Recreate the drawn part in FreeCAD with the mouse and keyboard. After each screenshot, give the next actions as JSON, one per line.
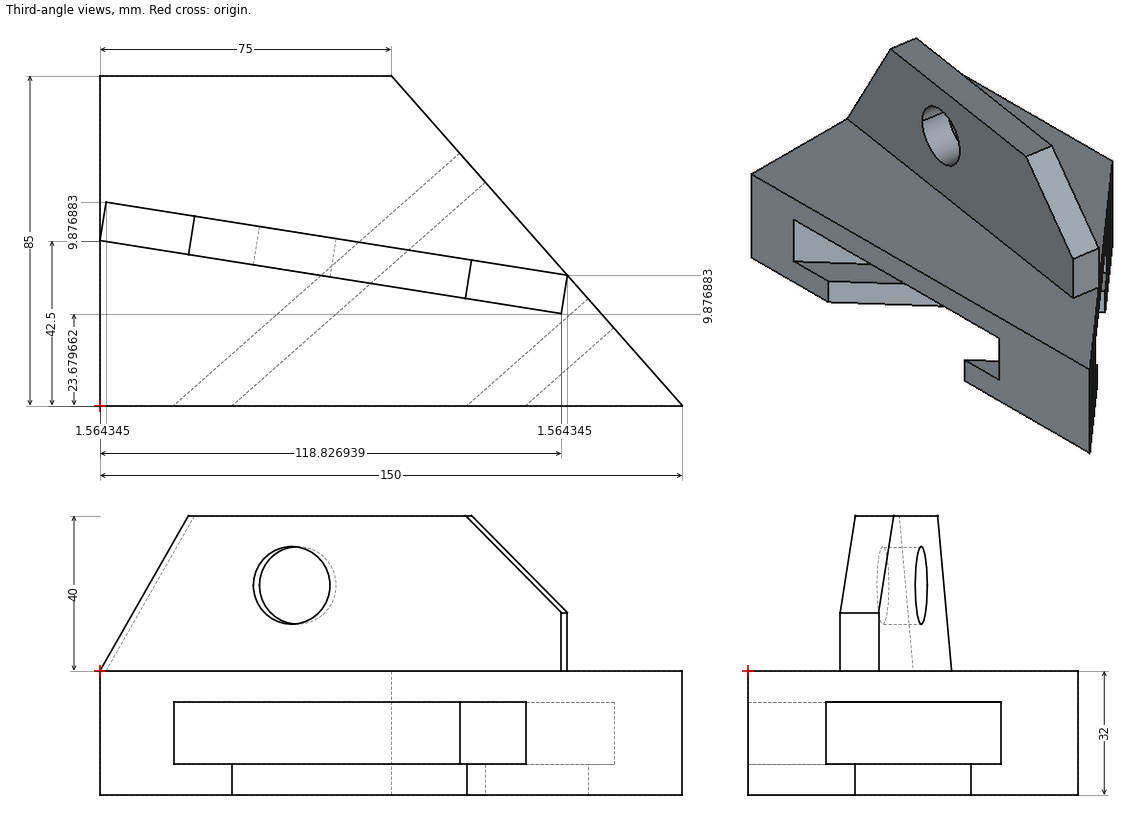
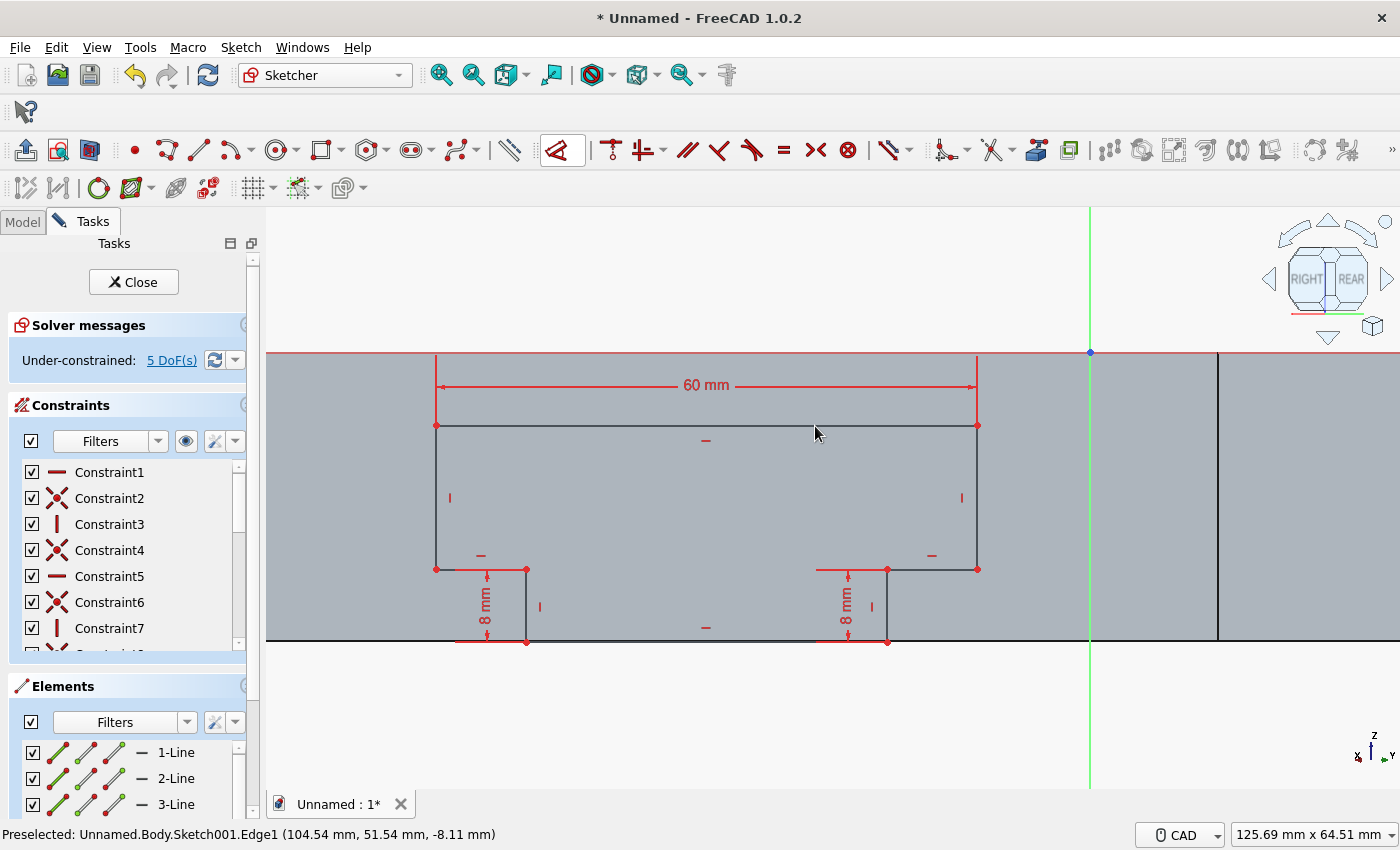
{"action": "left_click", "coordinate": [436, 469]}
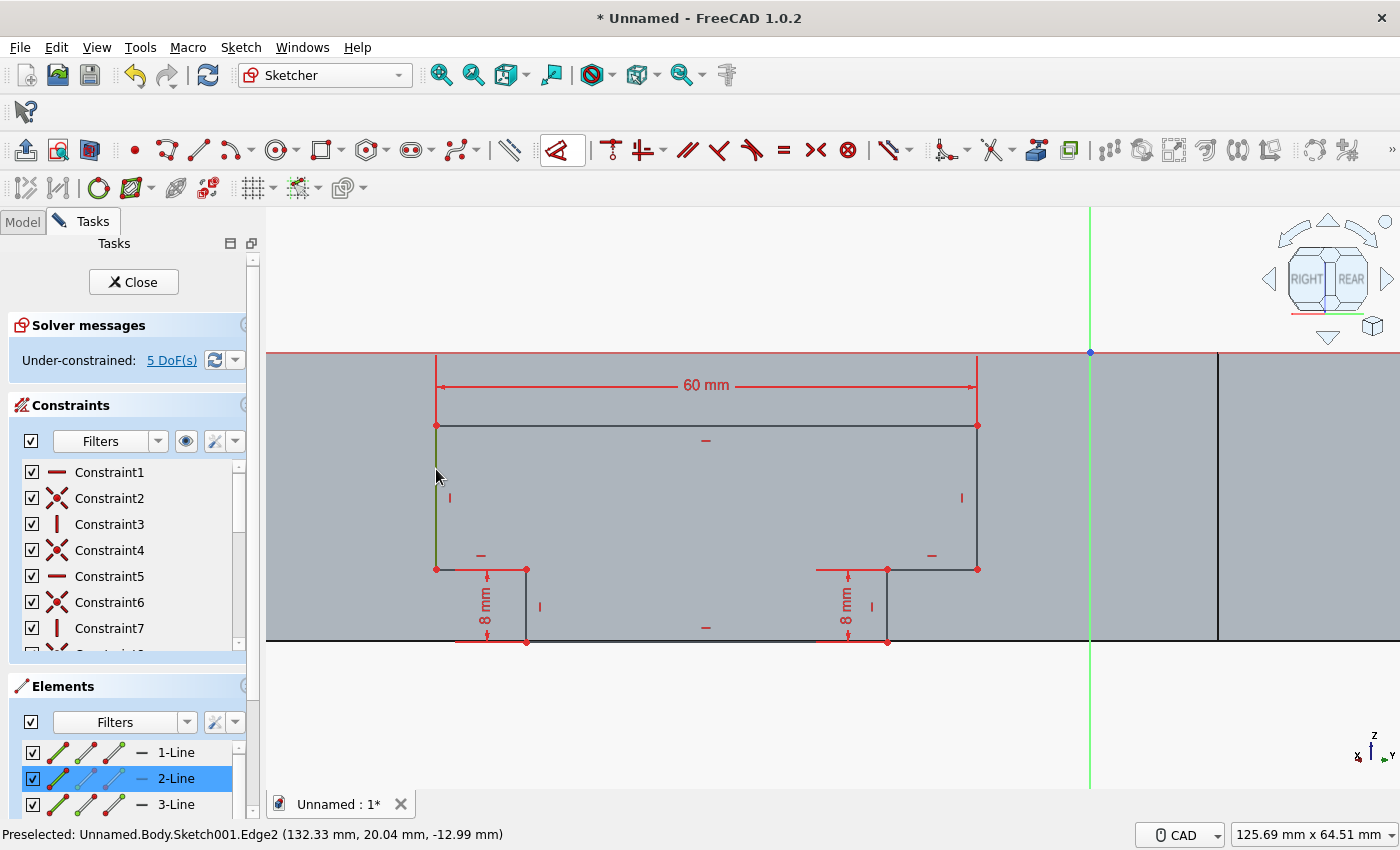
{"action": "key", "text": "i"}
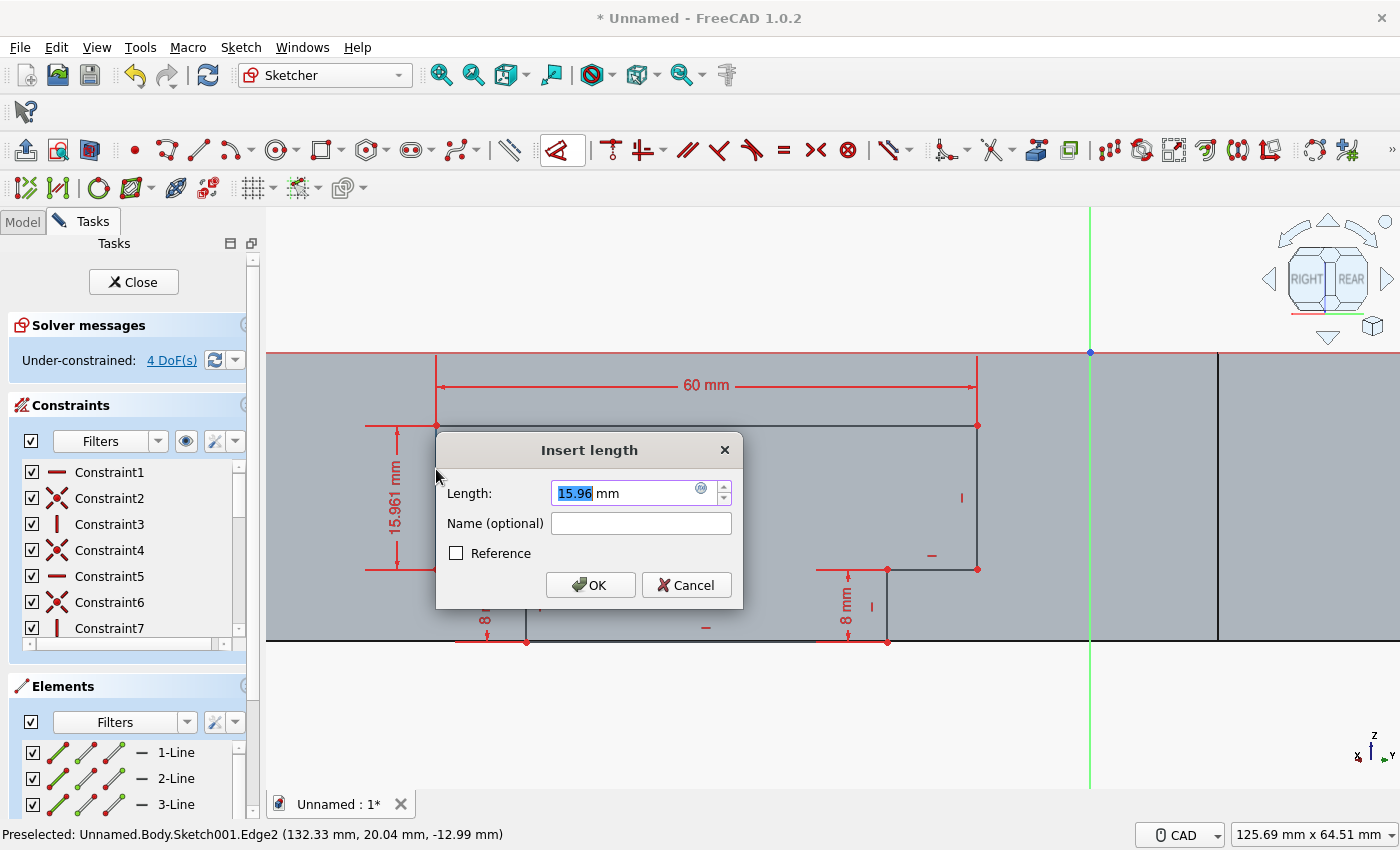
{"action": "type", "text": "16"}
{"action": "key", "text": "Return"}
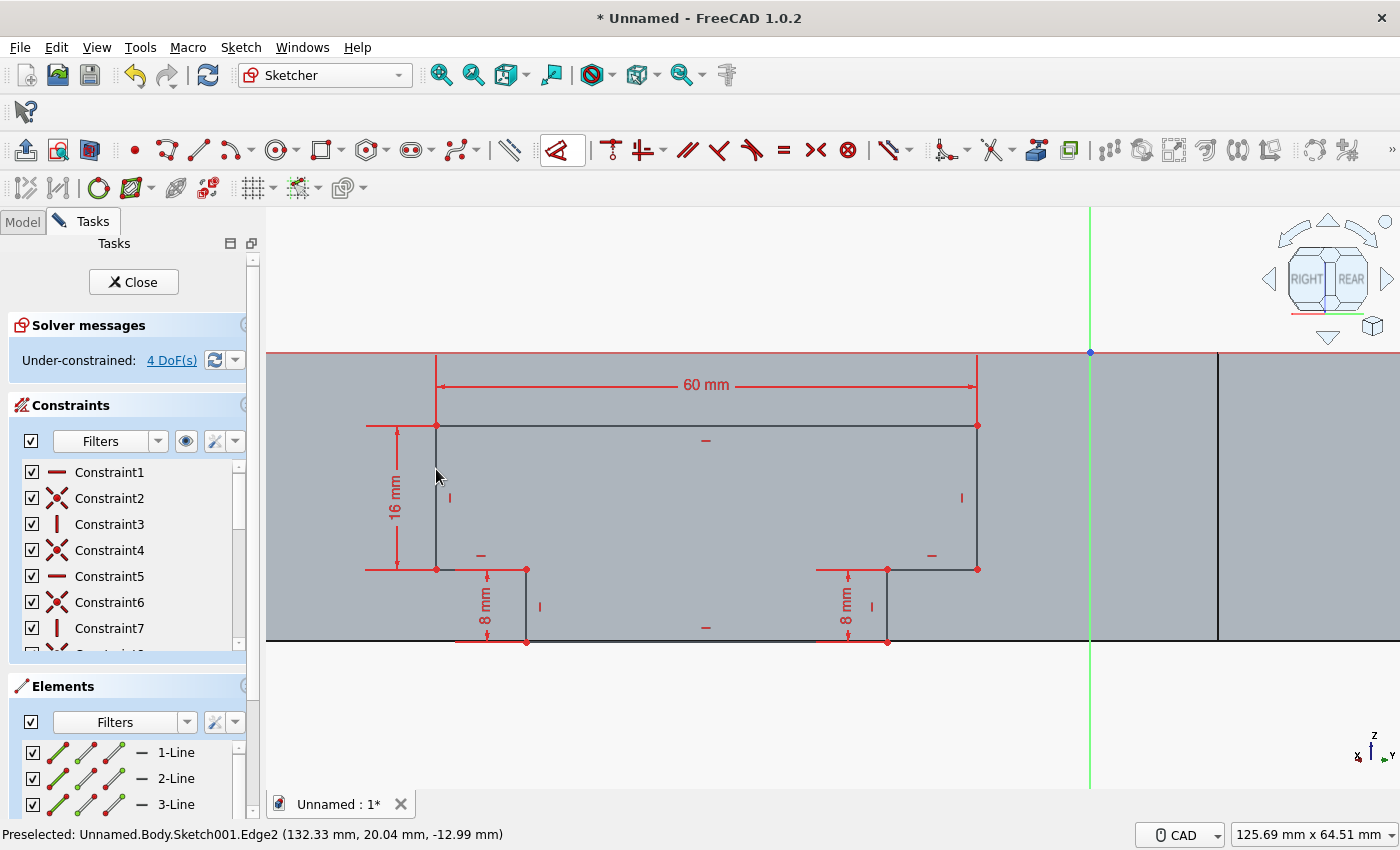
{"action": "left_click", "coordinate": [463, 570]}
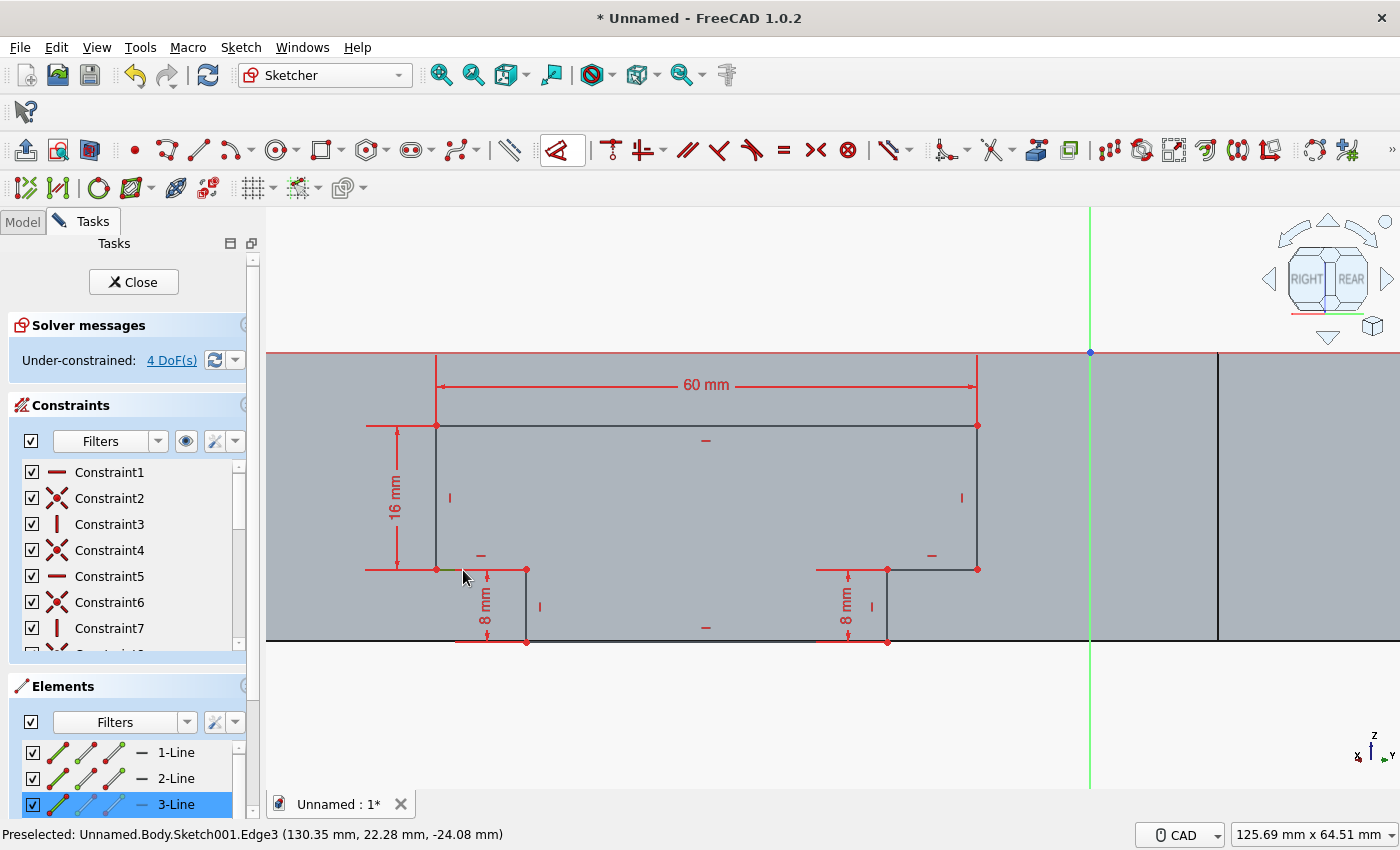
{"action": "key", "text": "l"}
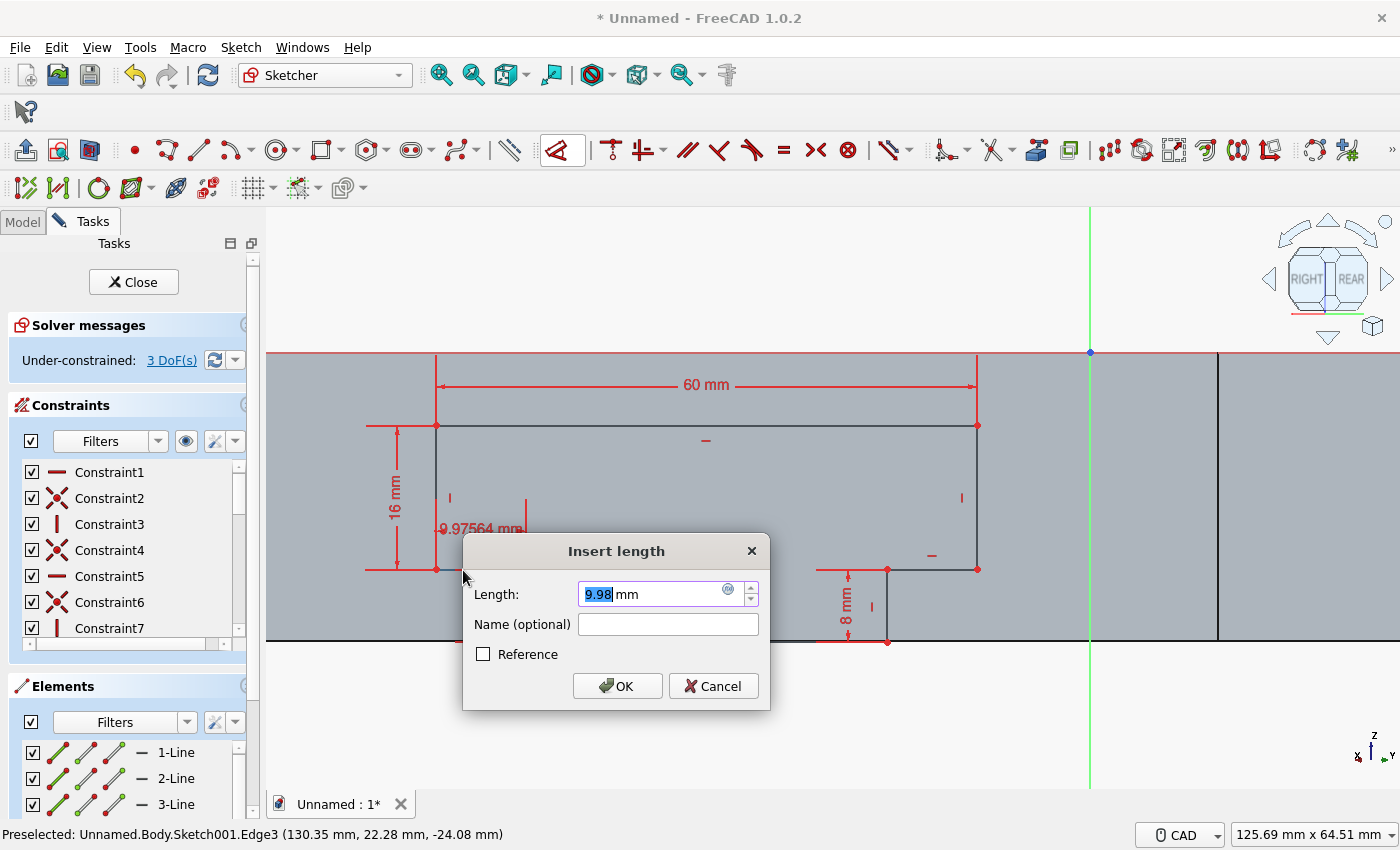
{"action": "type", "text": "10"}
{"action": "key", "text": "Return"}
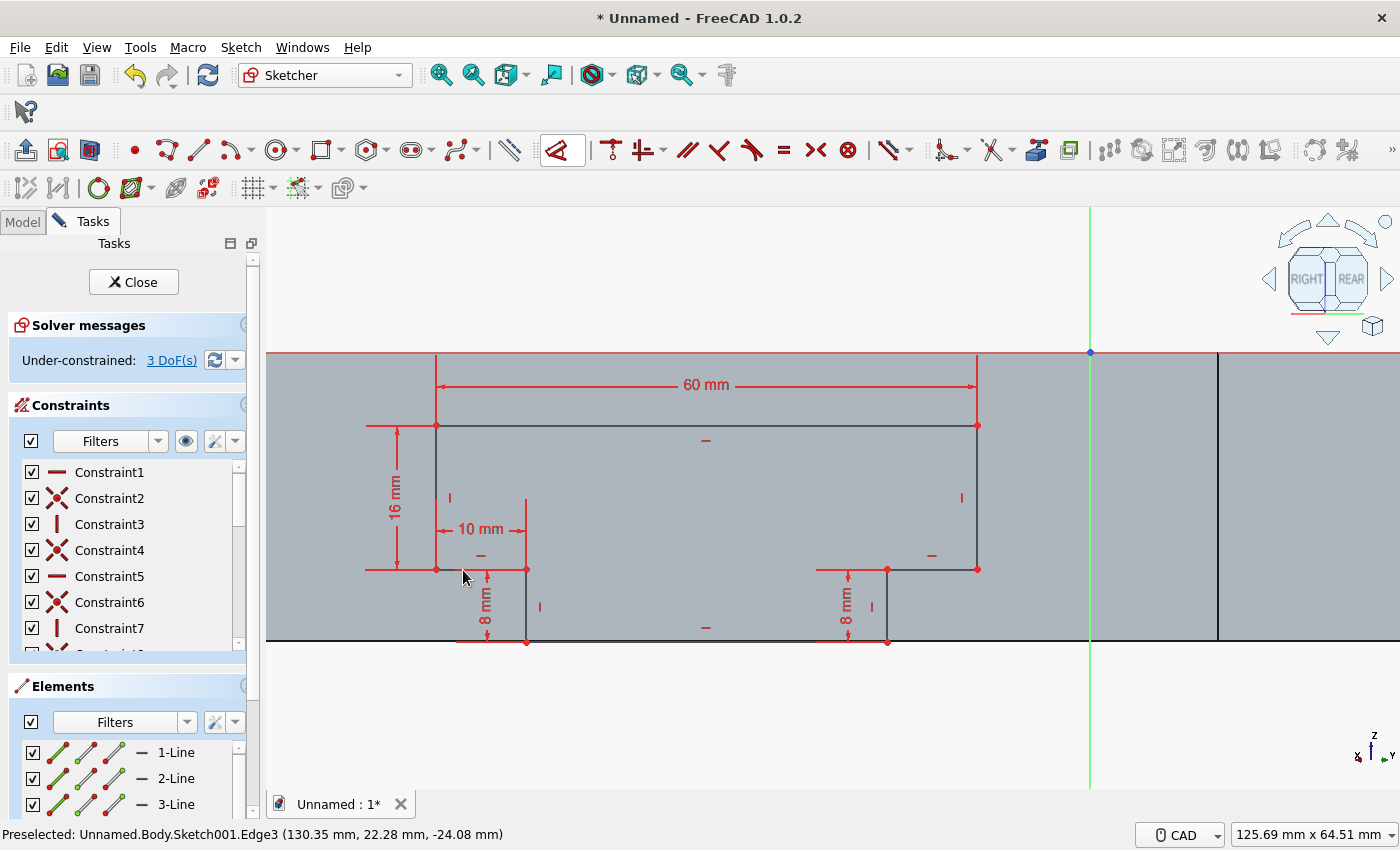
{"action": "left_click", "coordinate": [634, 642]}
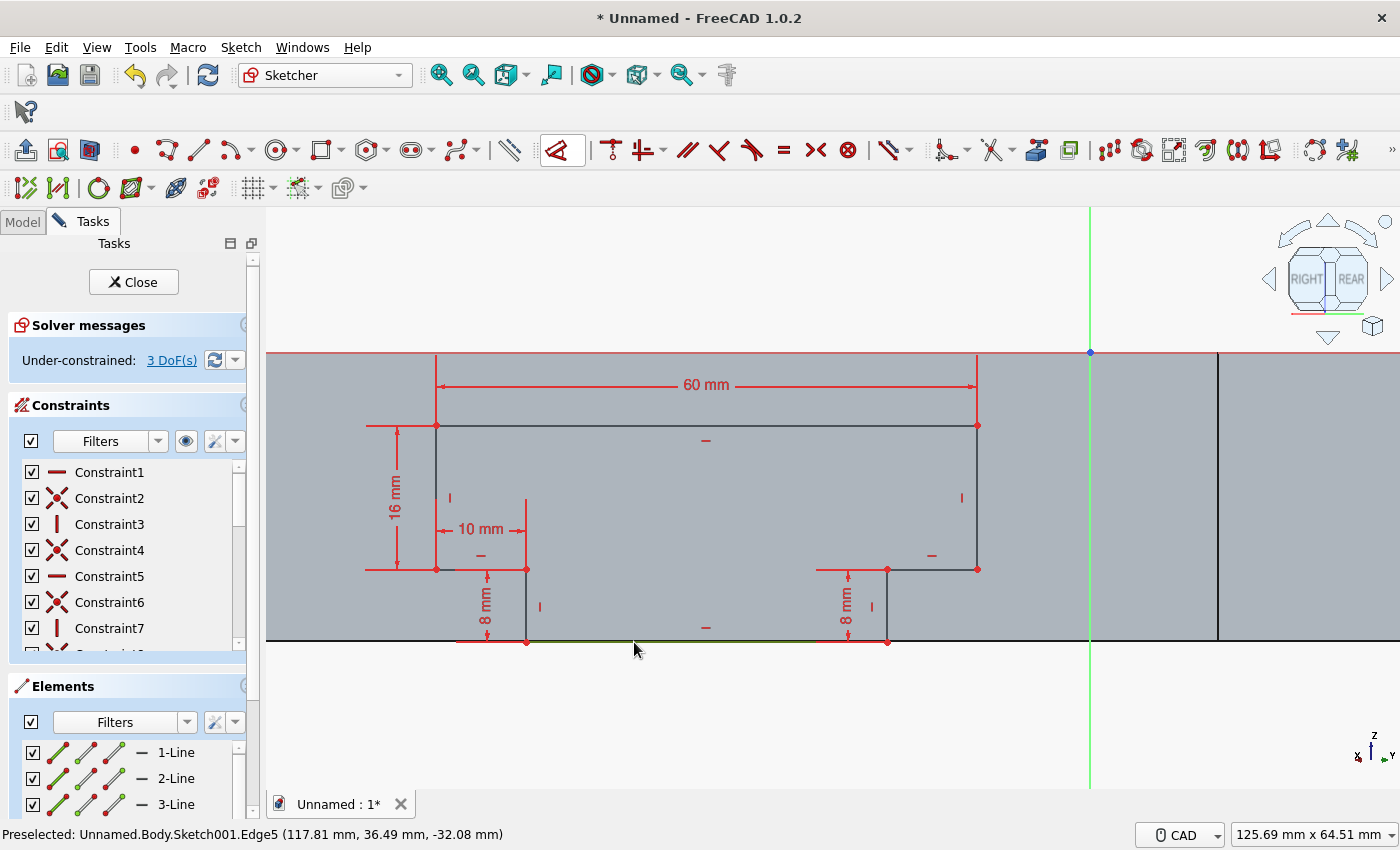
{"action": "key", "text": "l"}